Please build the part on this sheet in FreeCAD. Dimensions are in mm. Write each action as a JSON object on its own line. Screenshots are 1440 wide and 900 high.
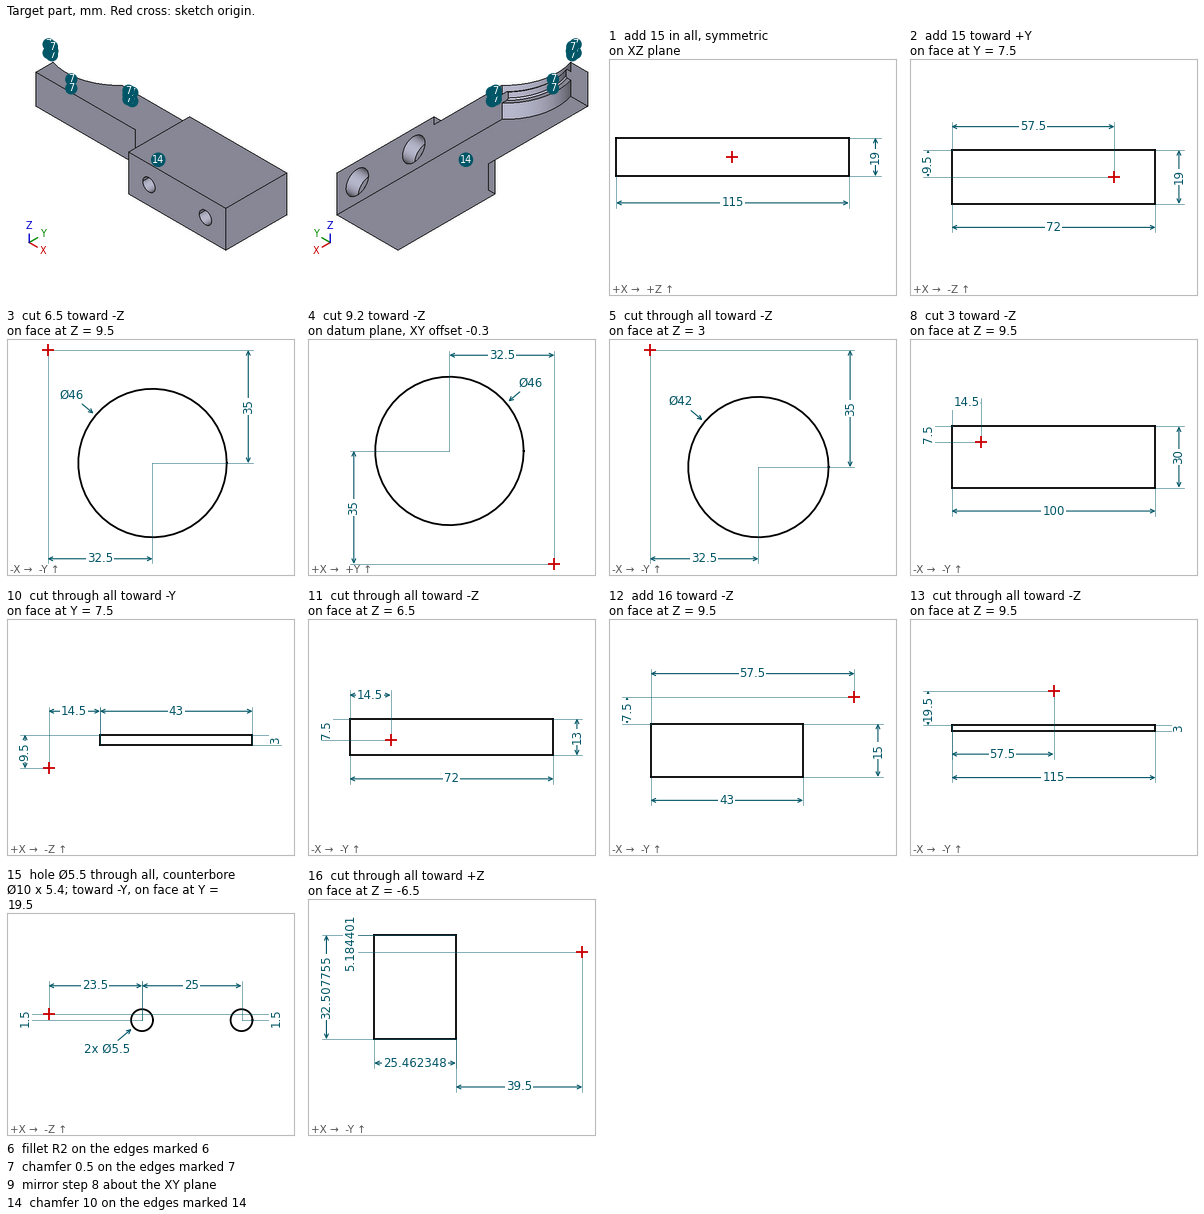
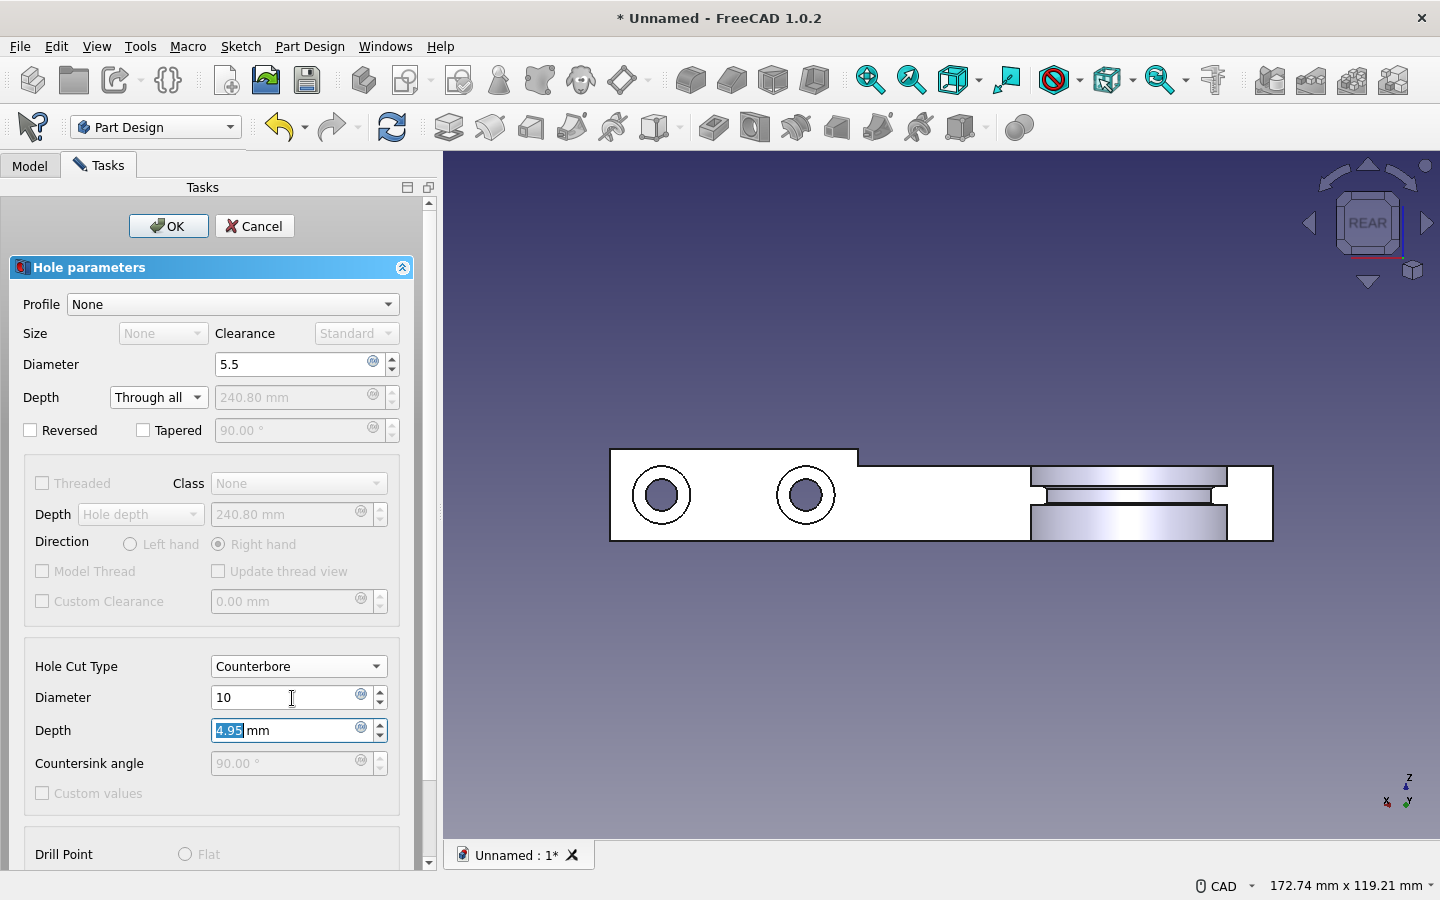
{"action": "type", "text": "5.4"}
{"action": "key", "text": "Tab"}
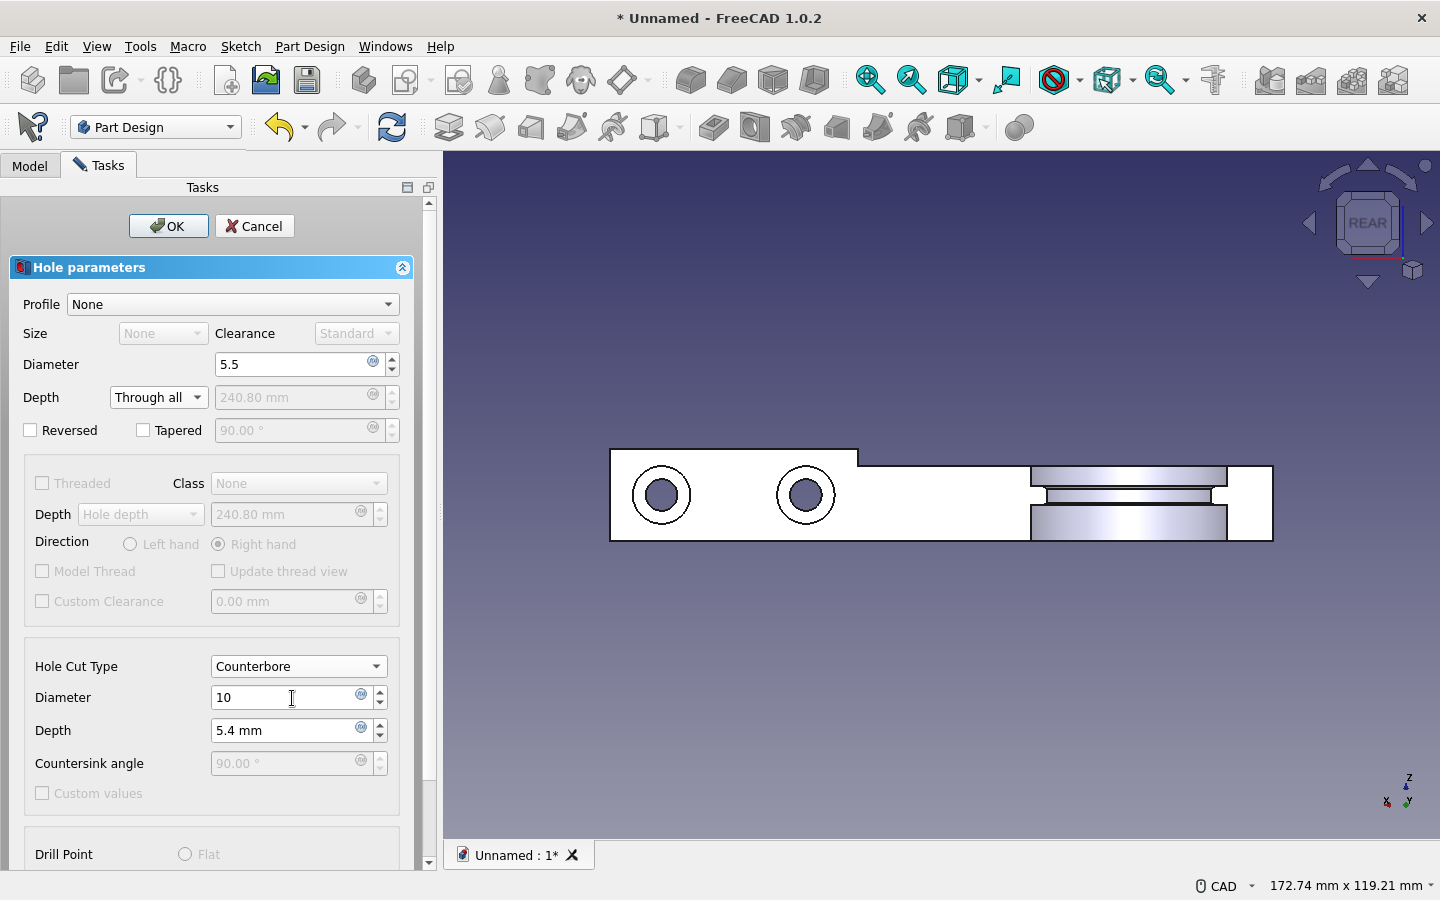
{"action": "left_click", "coordinate": [169, 226]}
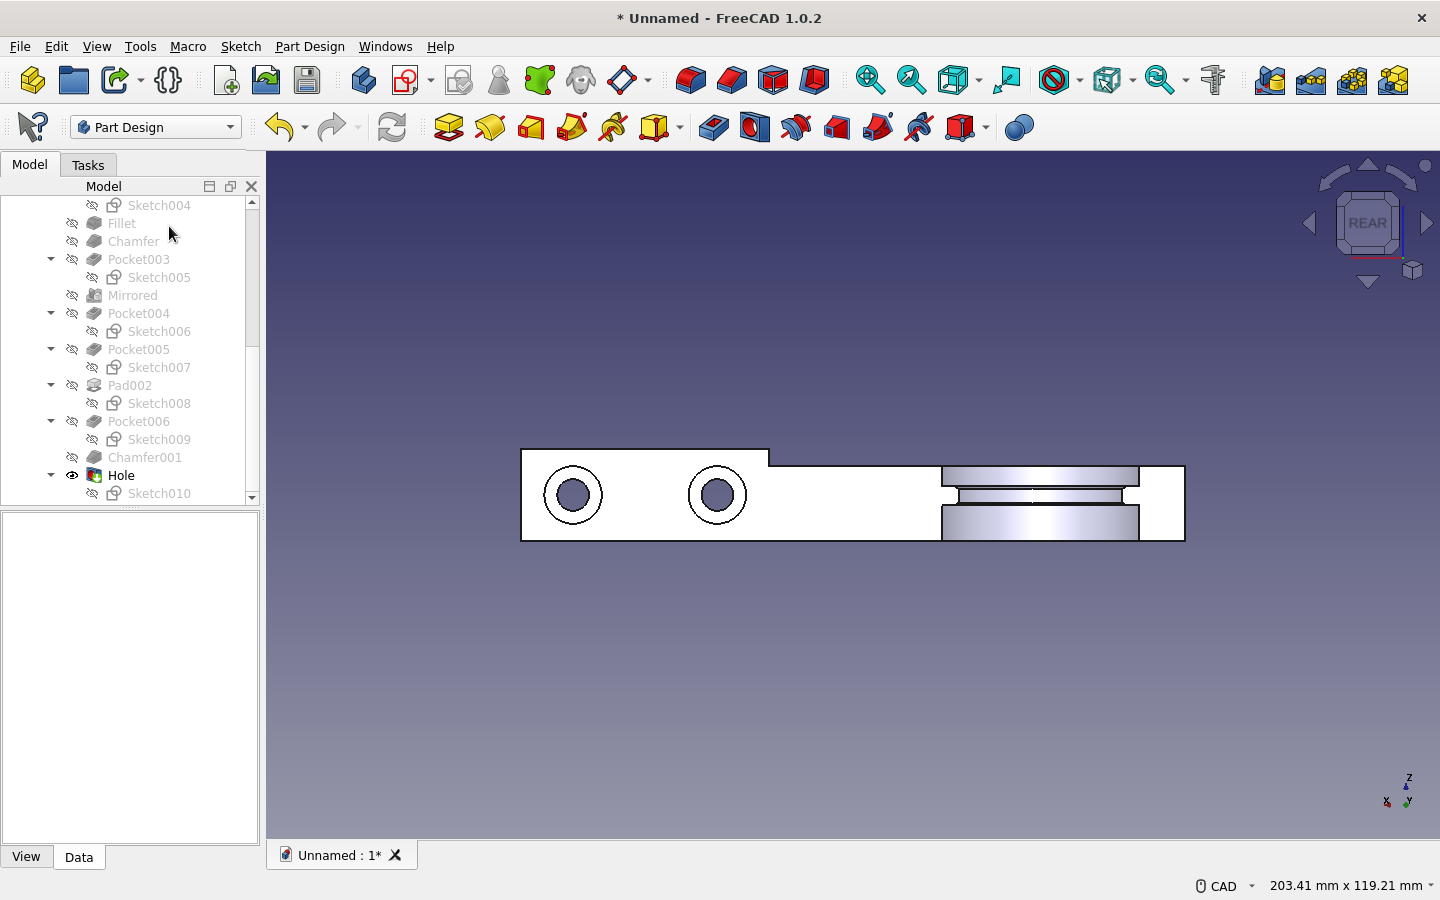
{"action": "key", "text": "5"}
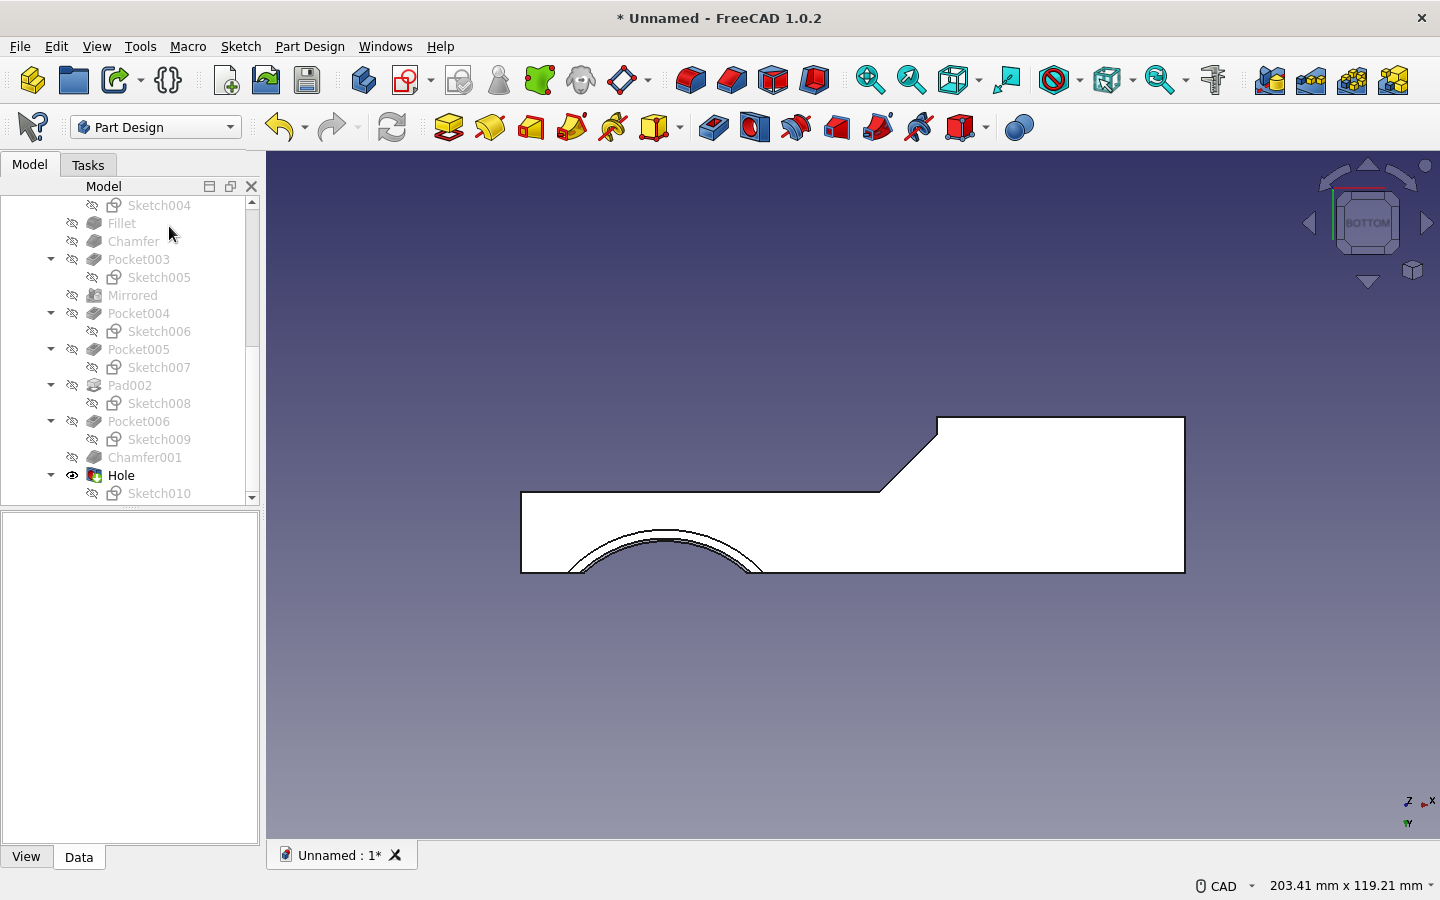
{"action": "left_click", "coordinate": [1043, 494]}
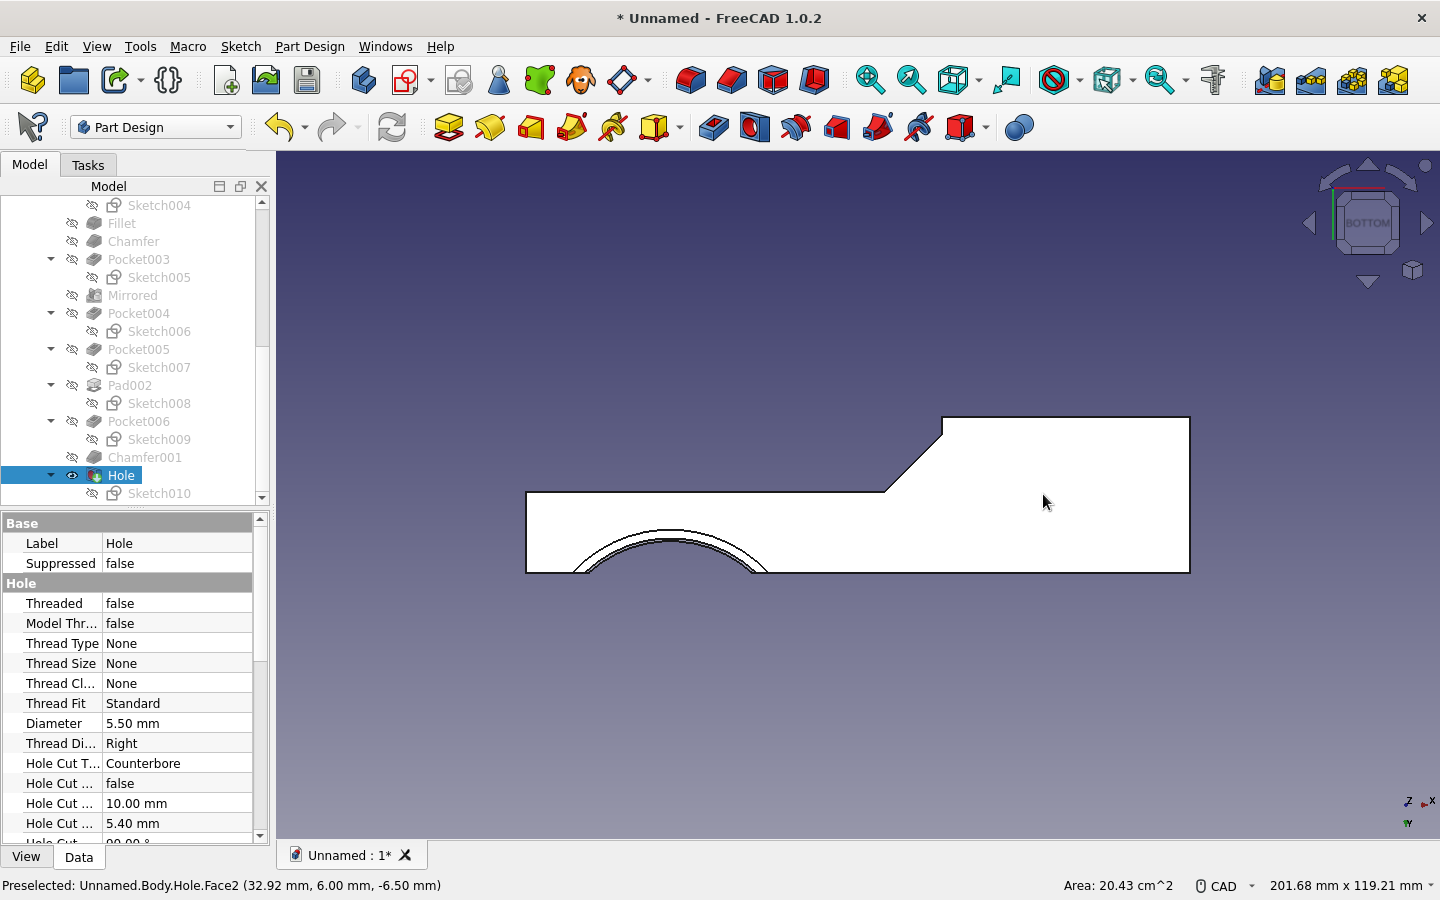
{"action": "left_click", "coordinate": [404, 80]}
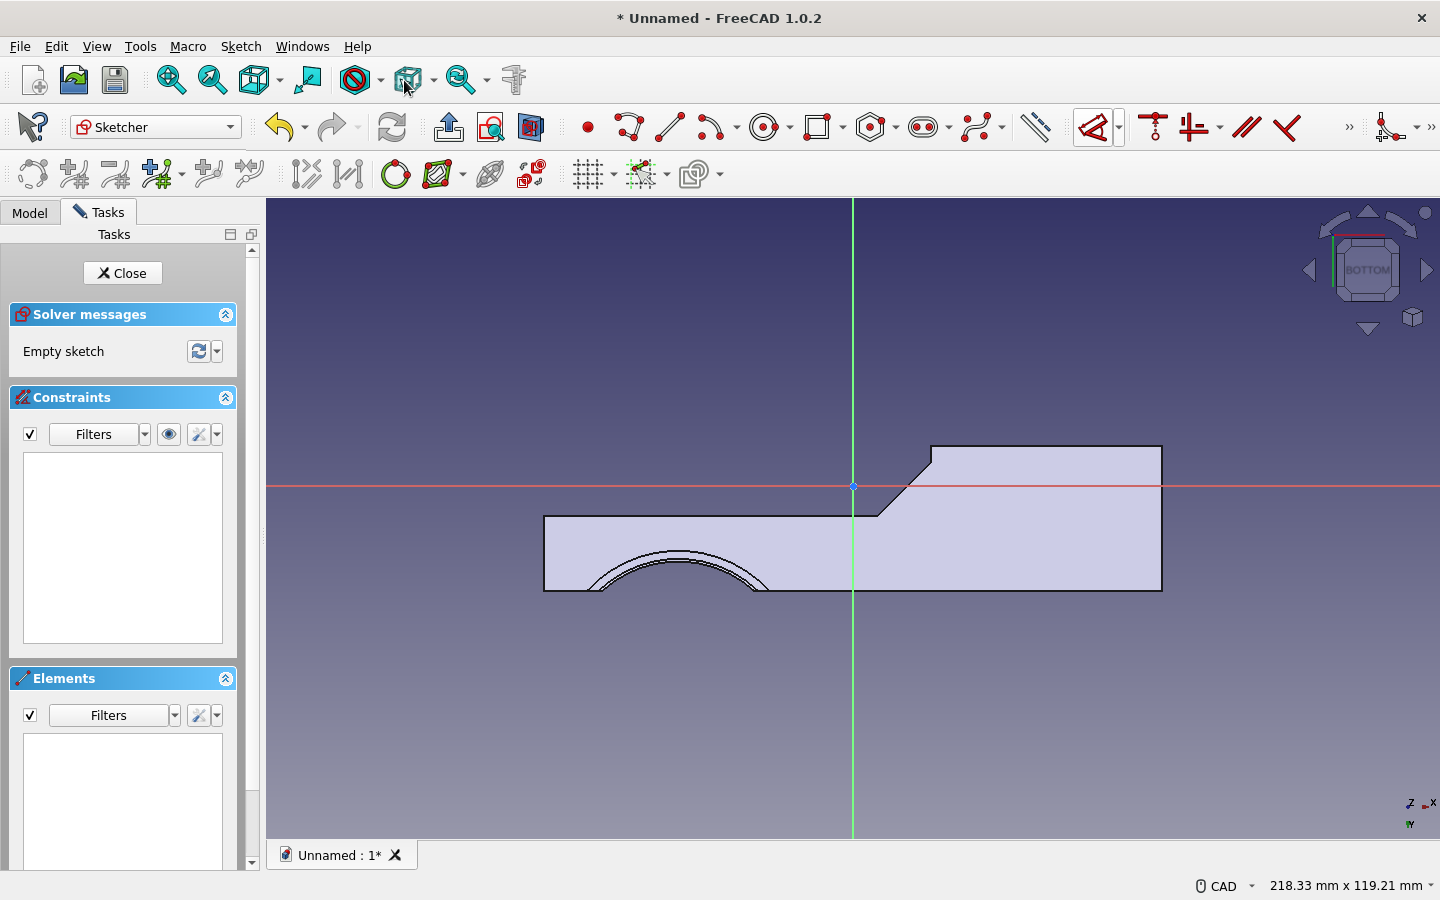
{"action": "scroll", "coordinate": [549, 579], "scroll_direction": "up", "scroll_amount": 3}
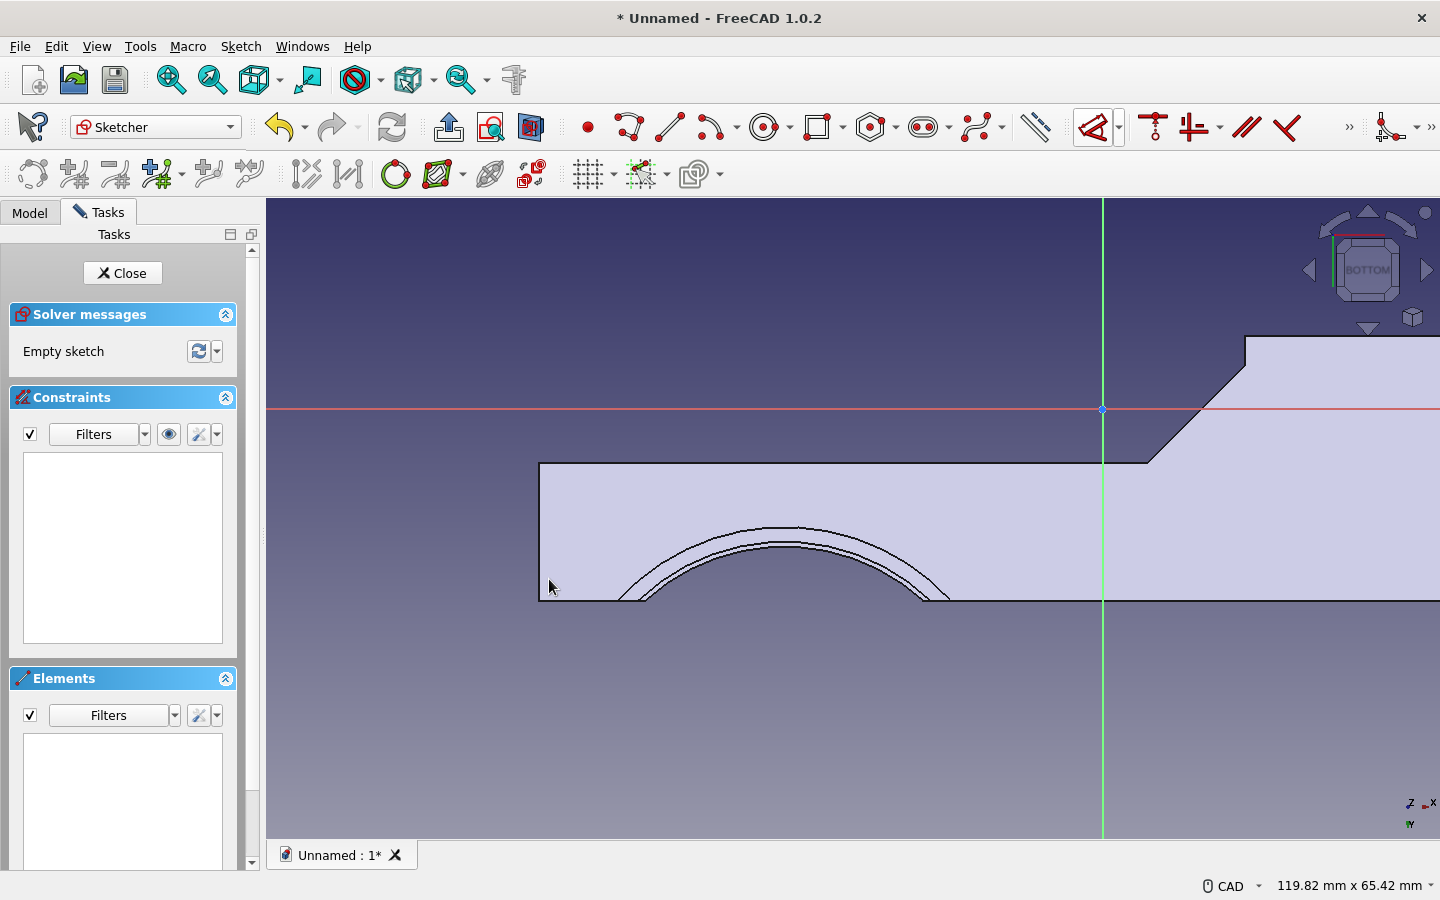
{"action": "left_click", "coordinate": [816, 128]}